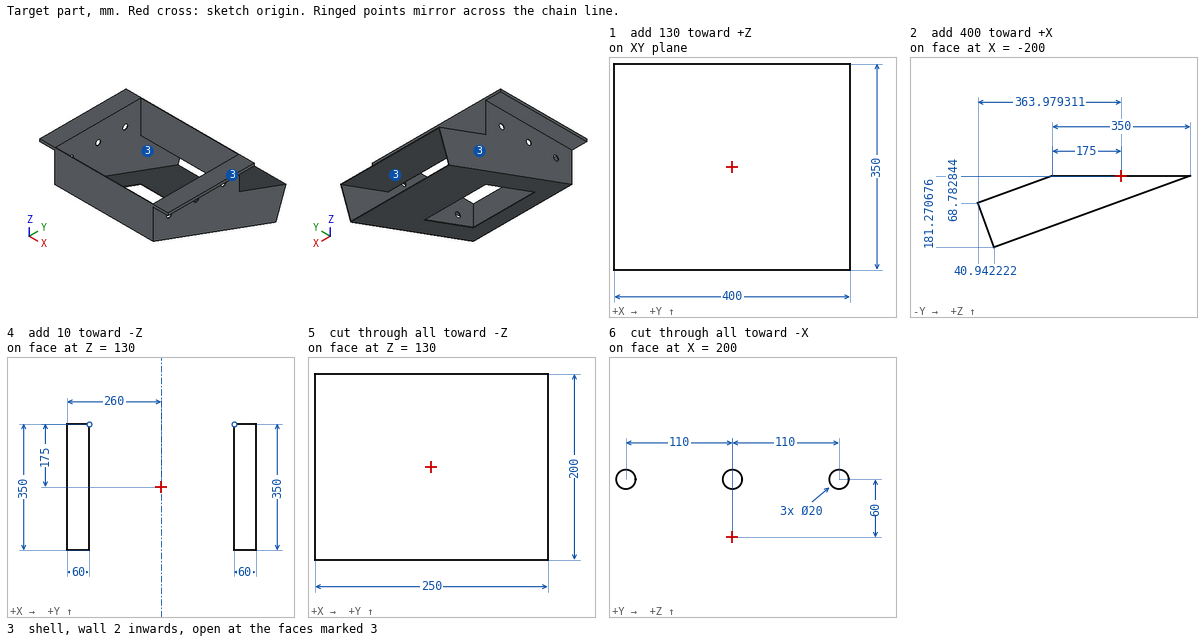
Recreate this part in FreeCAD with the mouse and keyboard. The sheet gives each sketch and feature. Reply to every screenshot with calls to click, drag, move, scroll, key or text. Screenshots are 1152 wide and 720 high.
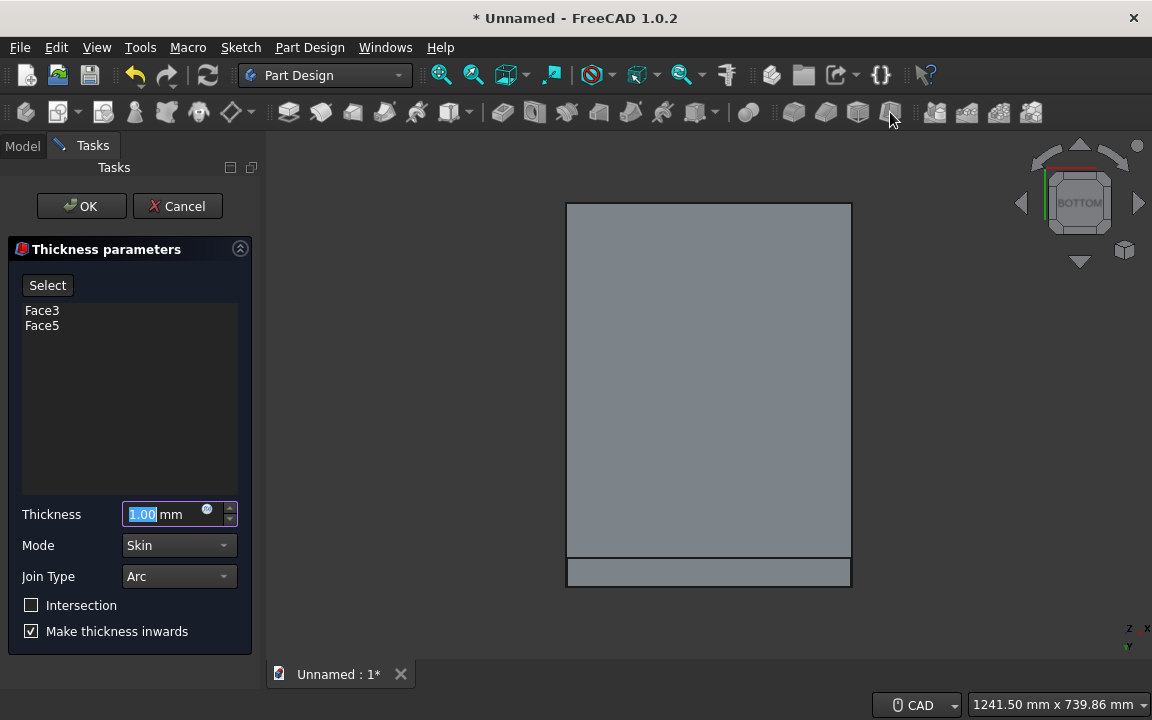
text(2)
key(Tab)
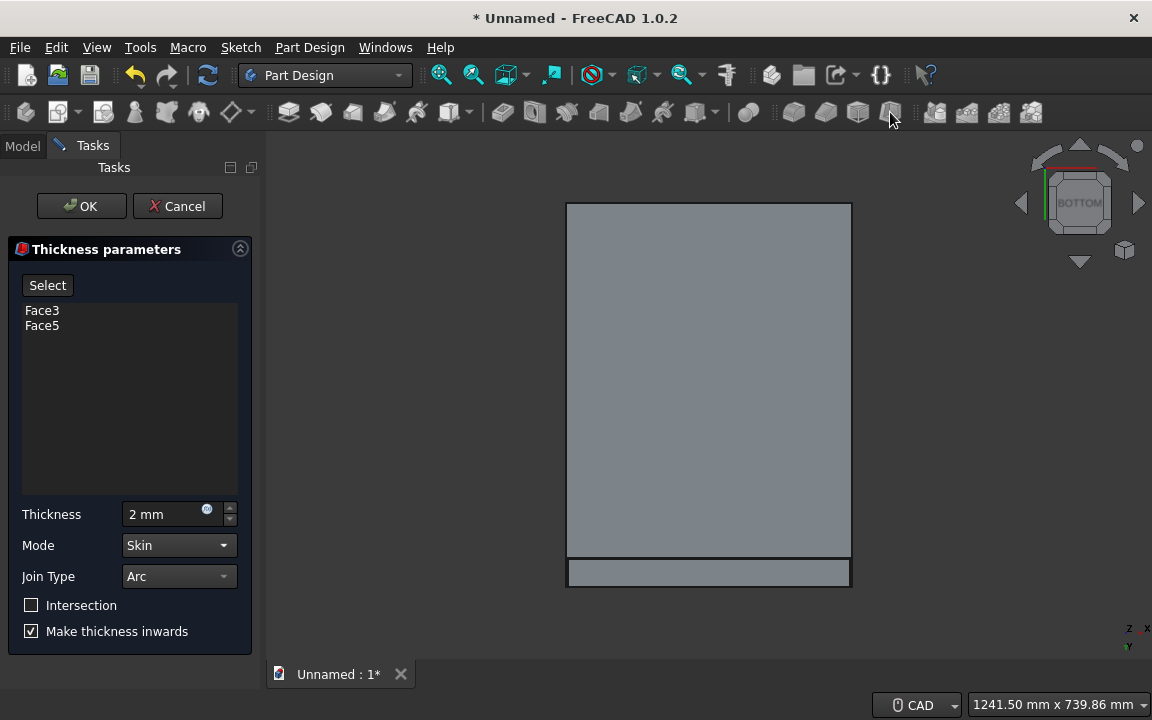
click(180, 576)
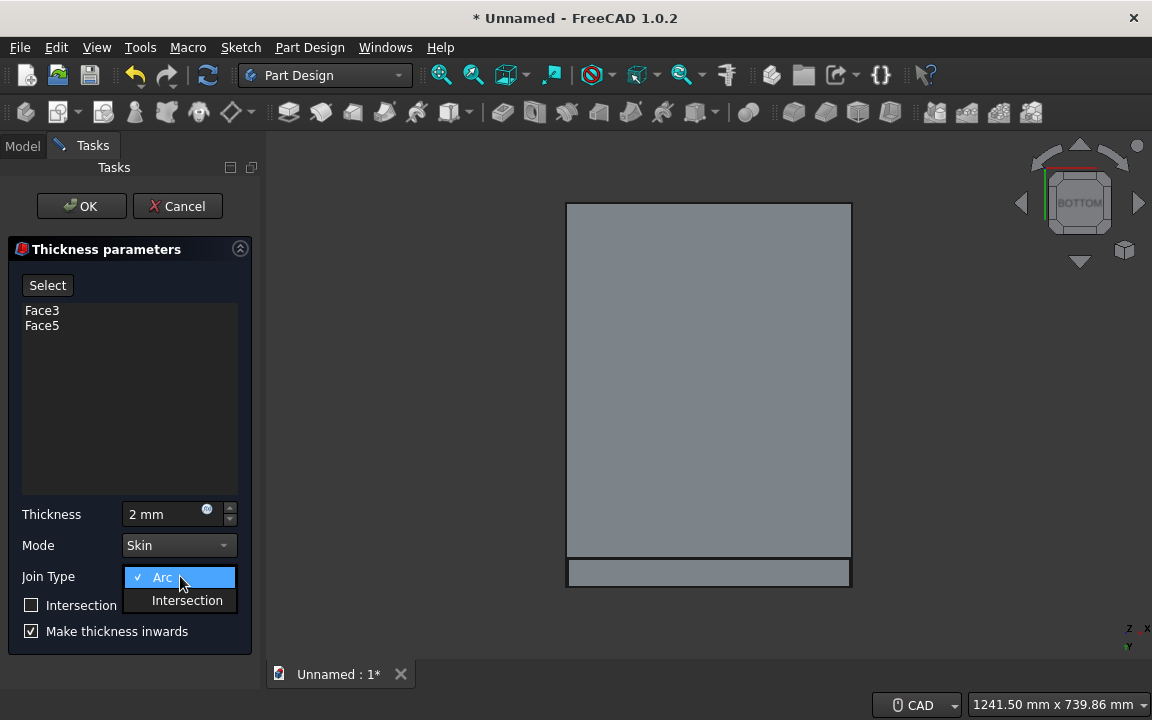
click(179, 600)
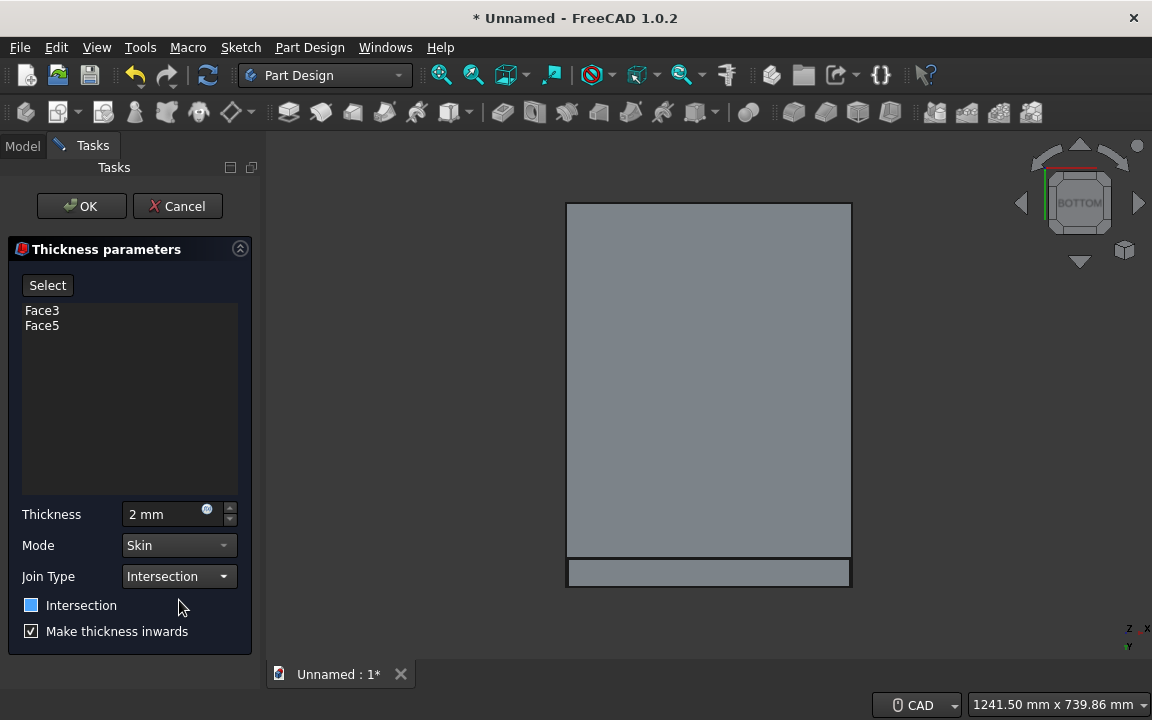
click(82, 206)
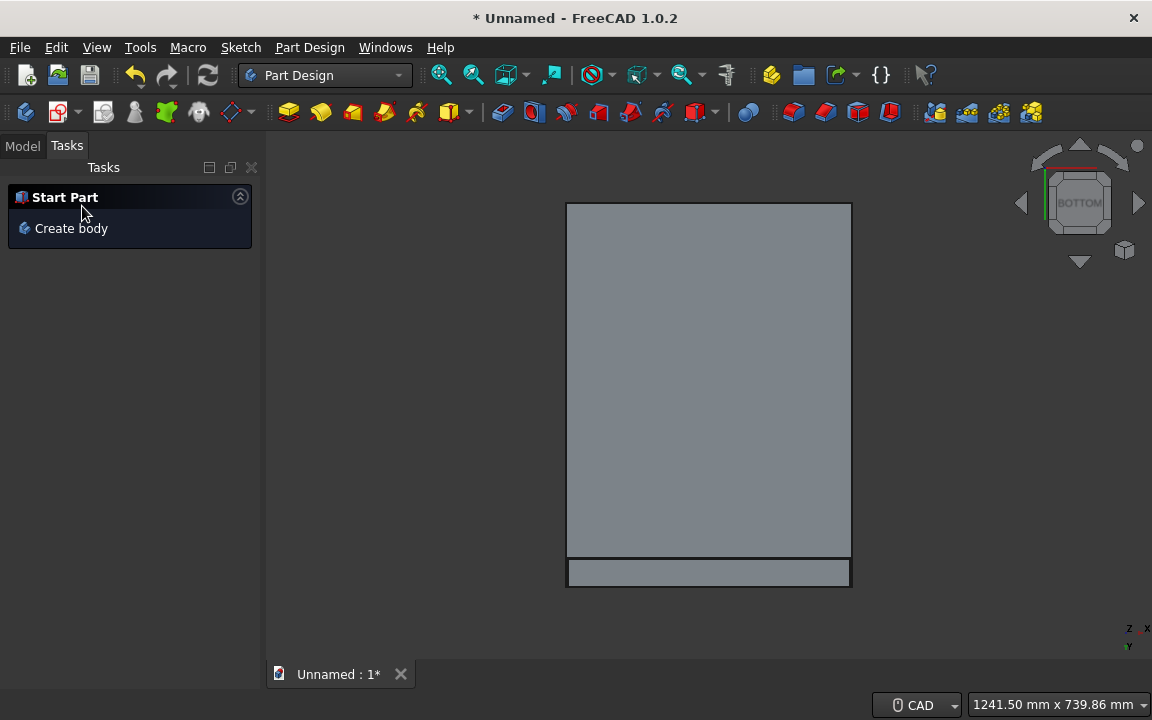
key(0)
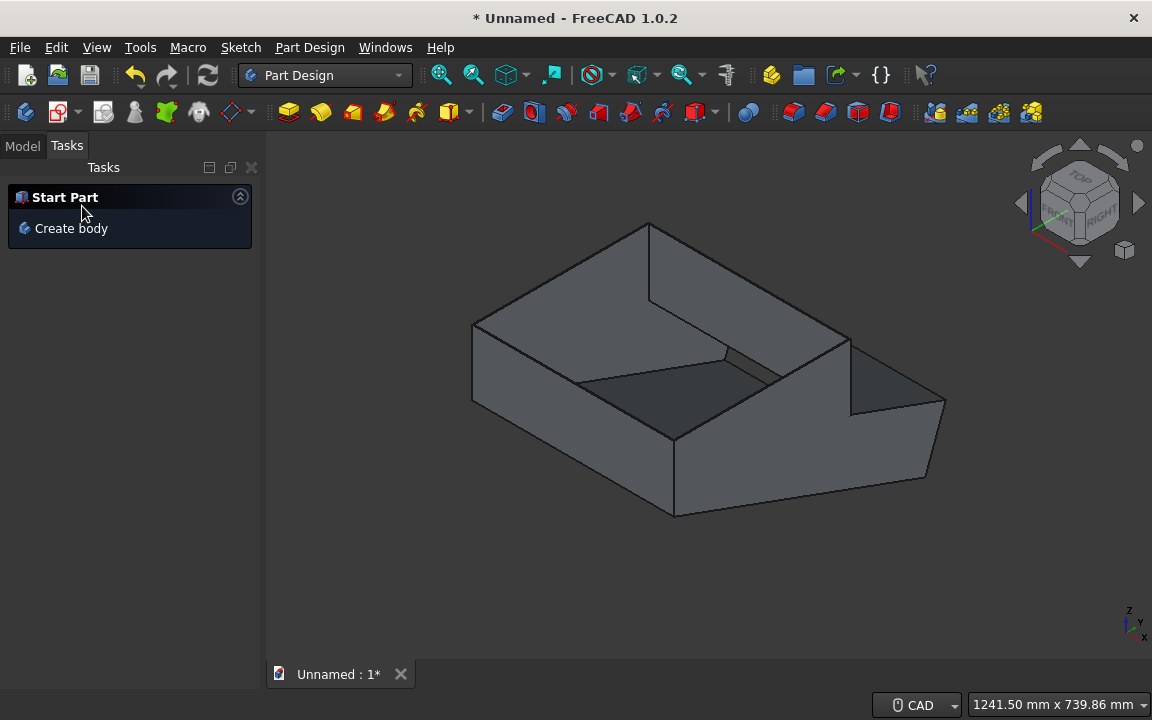
scroll(791, 372, up, 15)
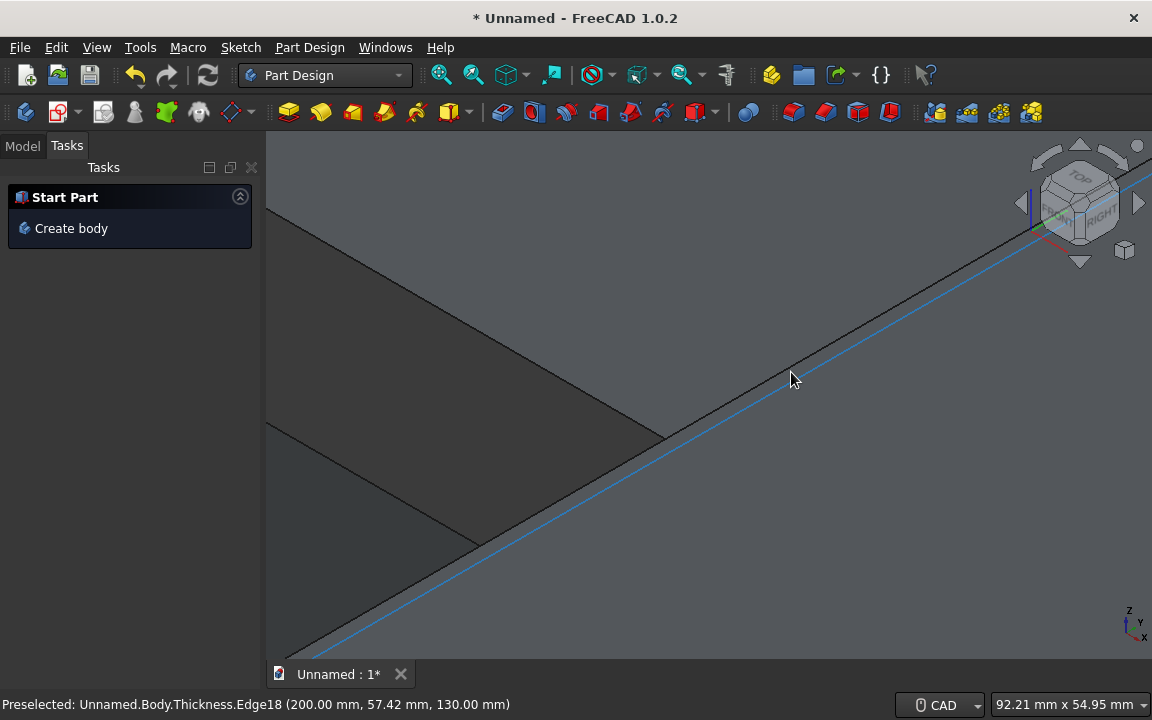
click(442, 76)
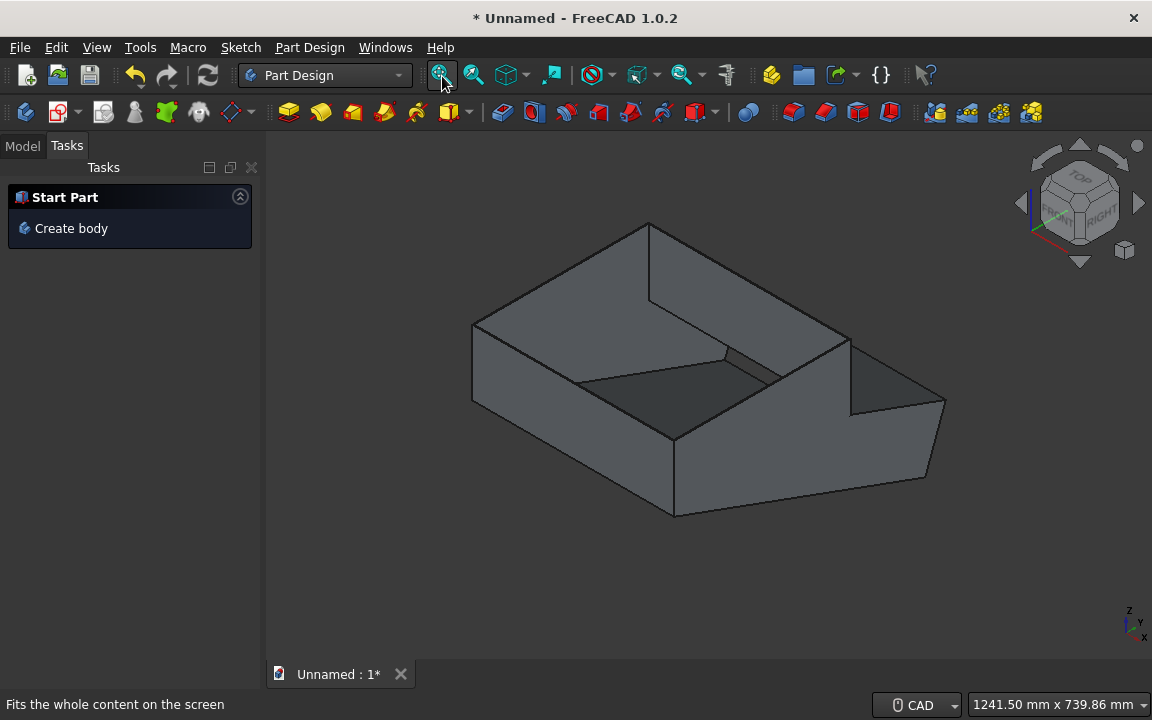
key(2)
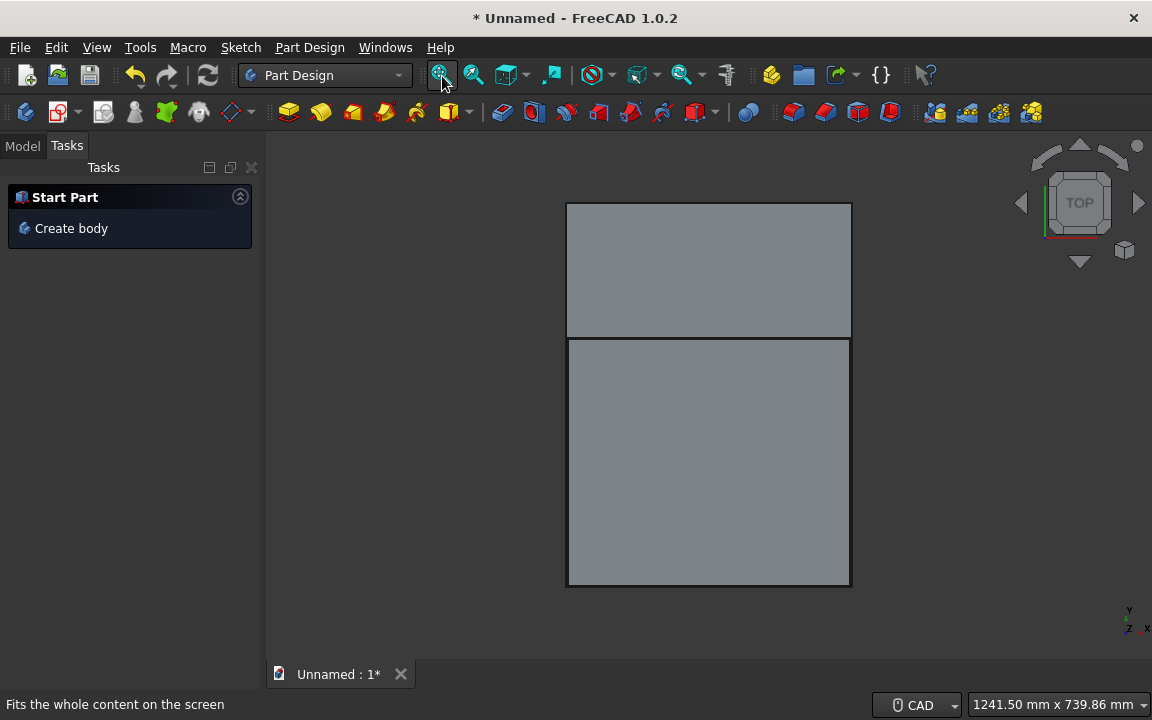
scroll(851, 420, up, 15)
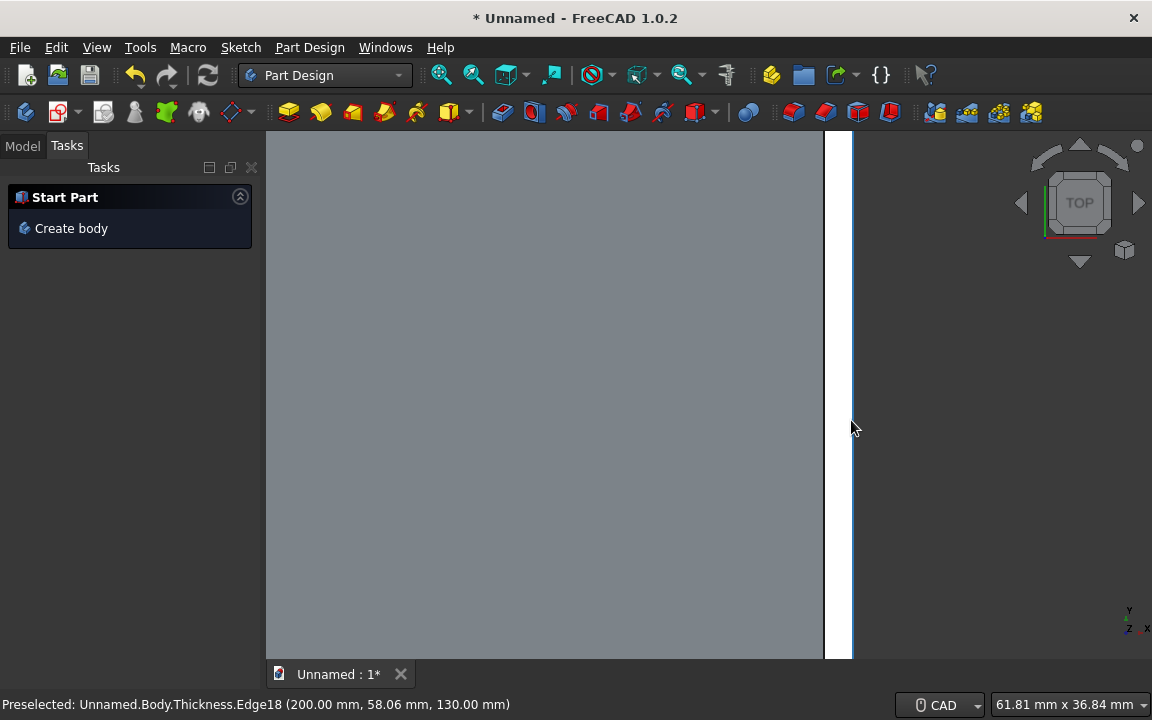
click(843, 434)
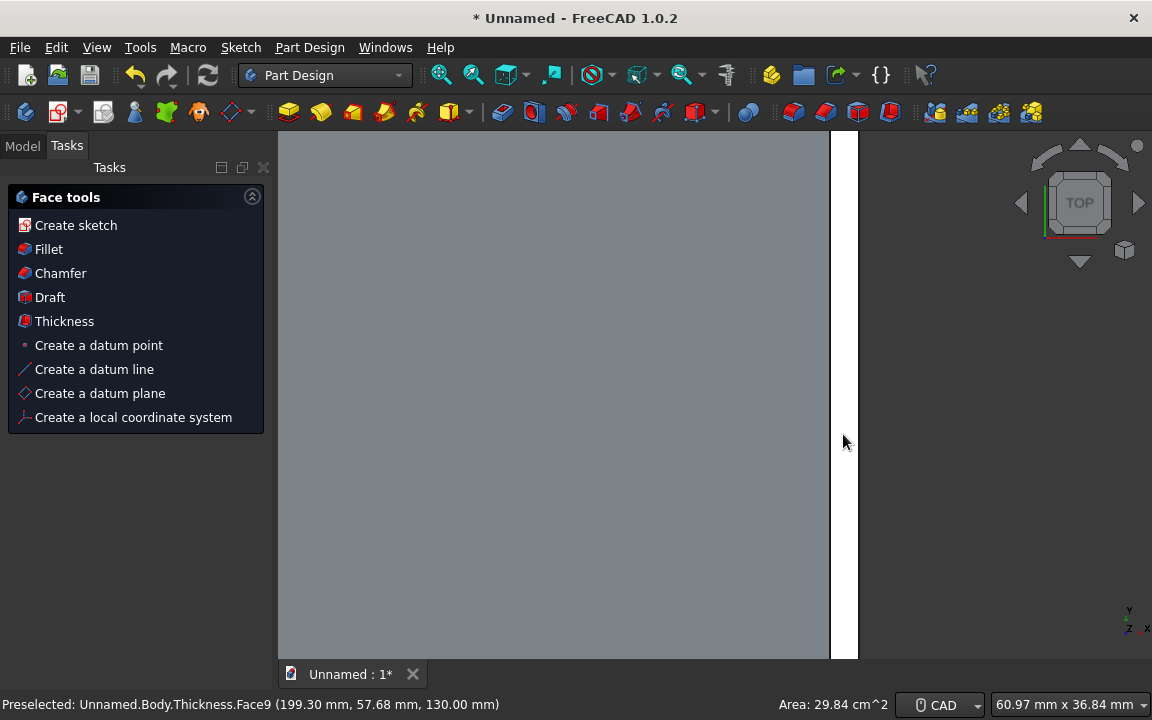
click(58, 112)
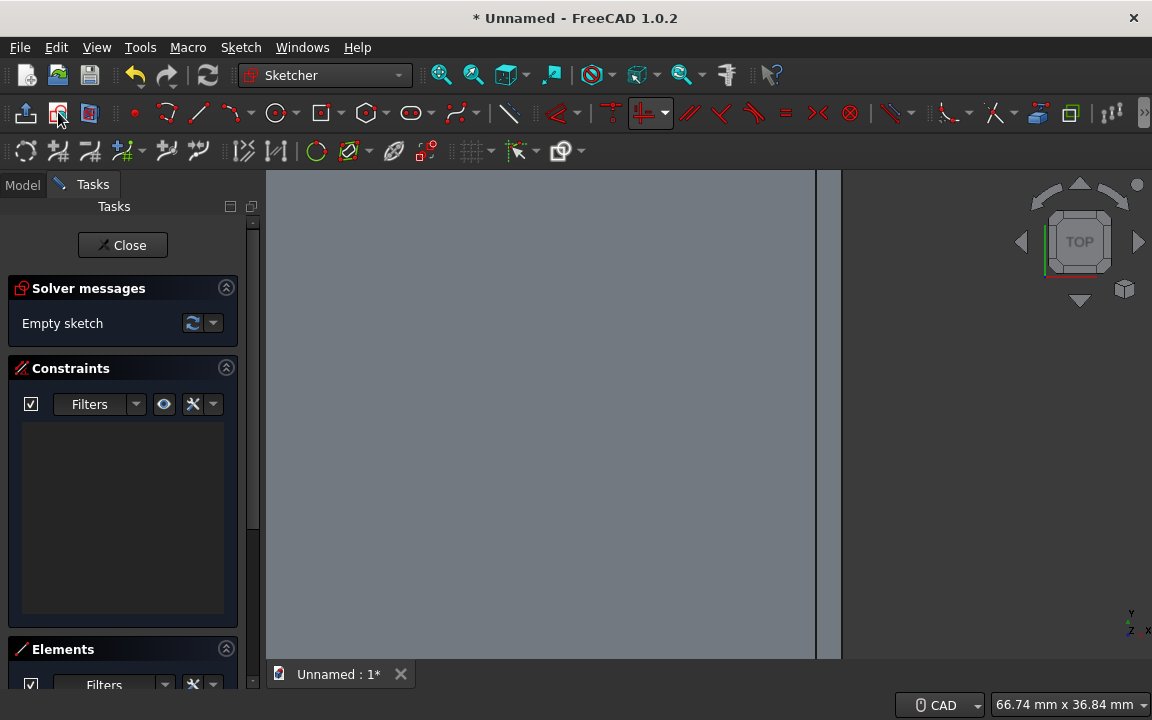
scroll(799, 363, down, 14)